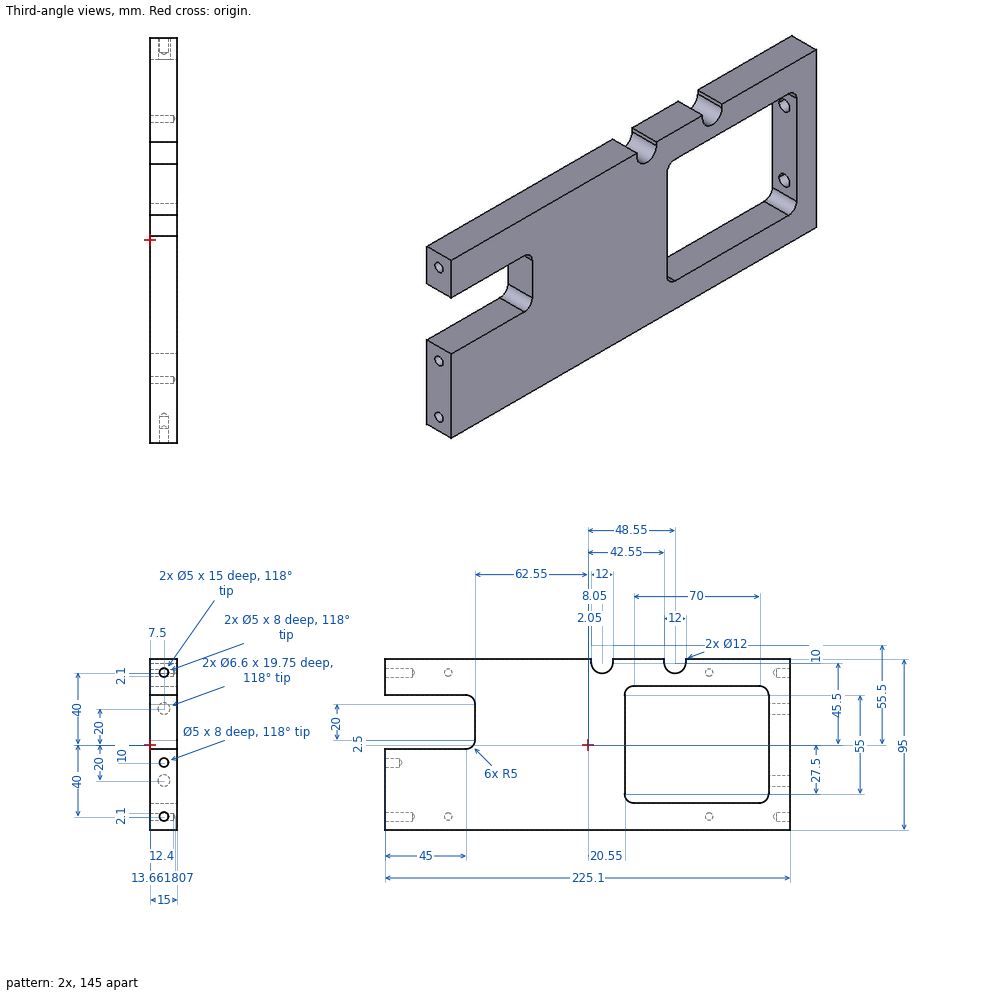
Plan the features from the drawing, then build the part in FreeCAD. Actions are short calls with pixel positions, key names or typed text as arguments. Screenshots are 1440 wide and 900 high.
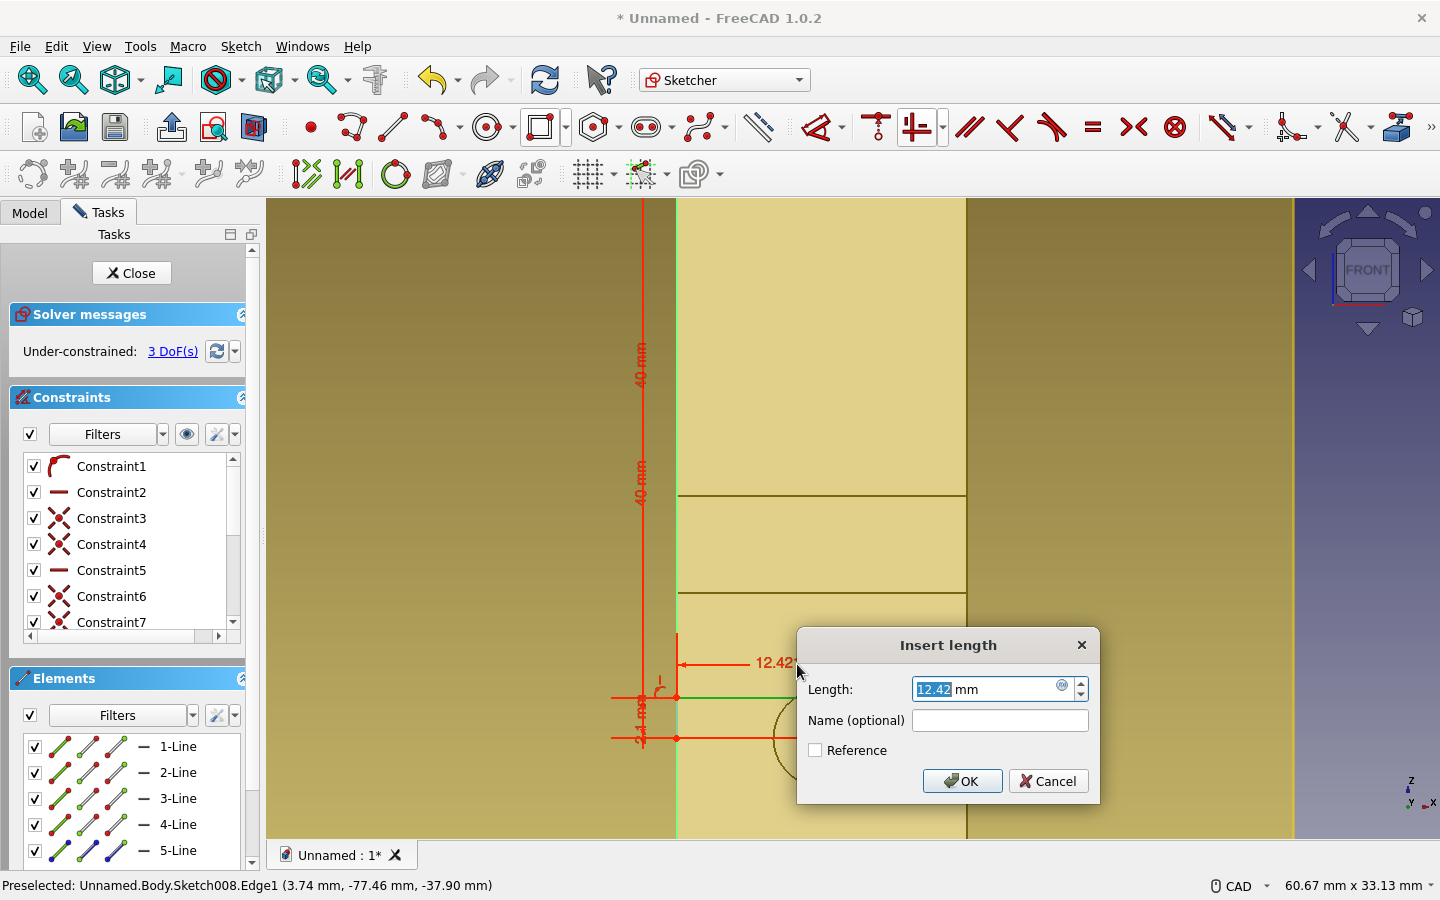
text(12.4)
key(Return)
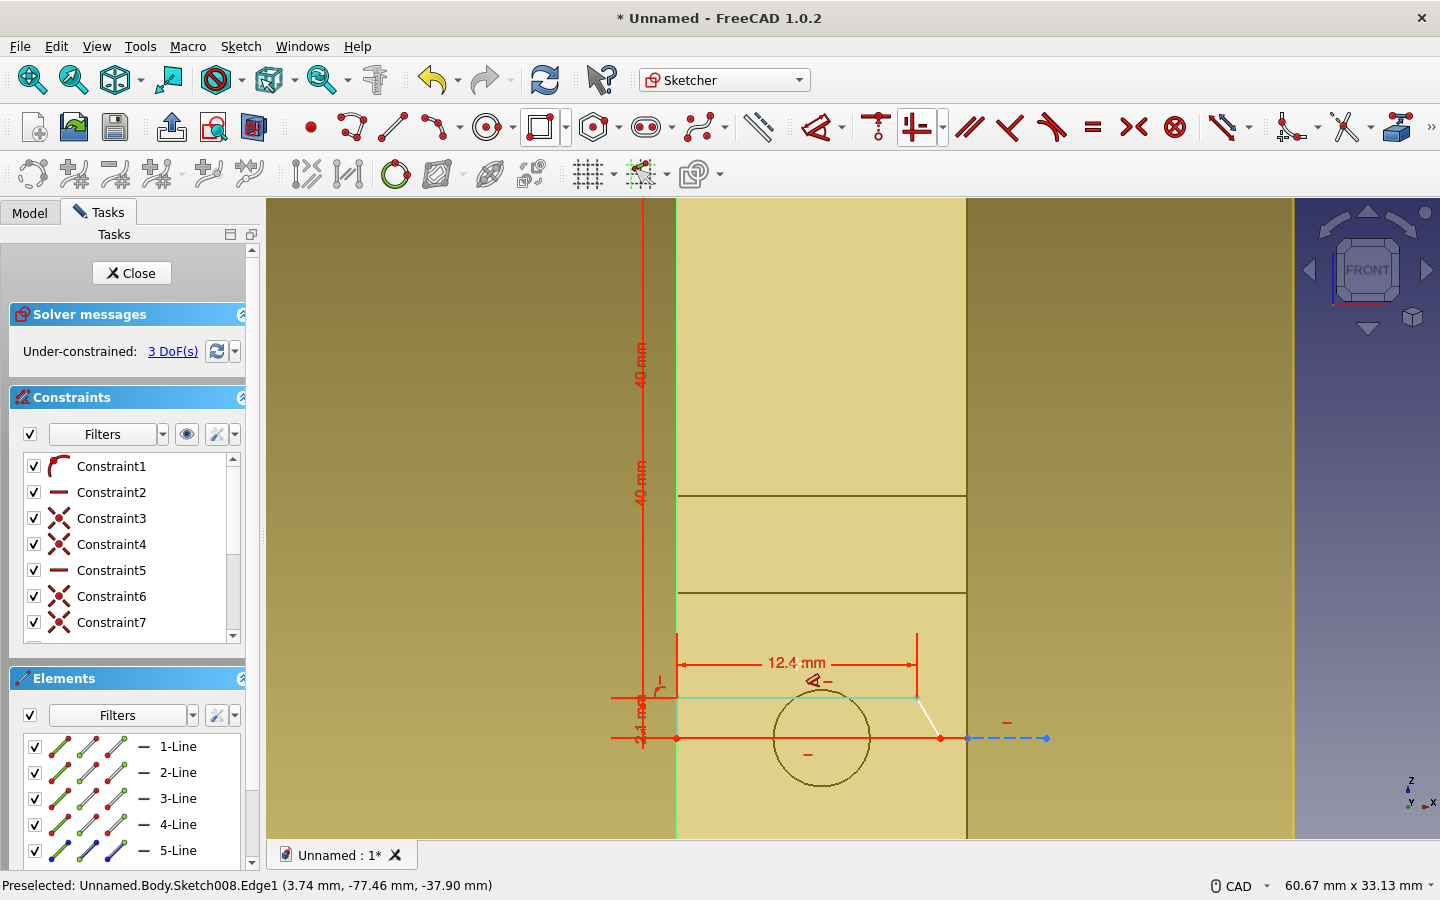
click(861, 738)
click(809, 772)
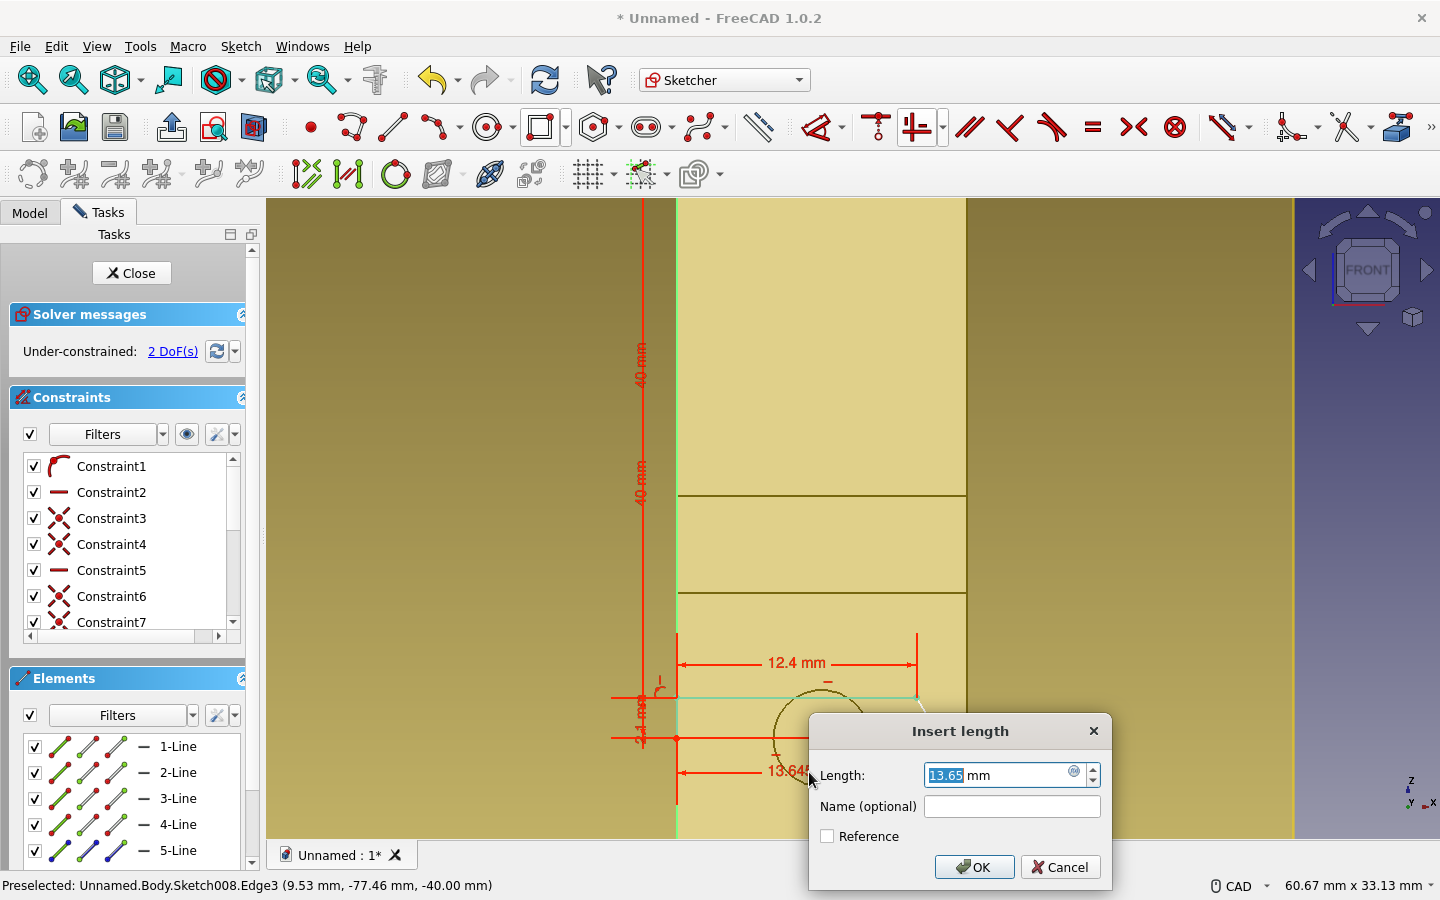
text(13.661807)
key(Return)
key(Escape)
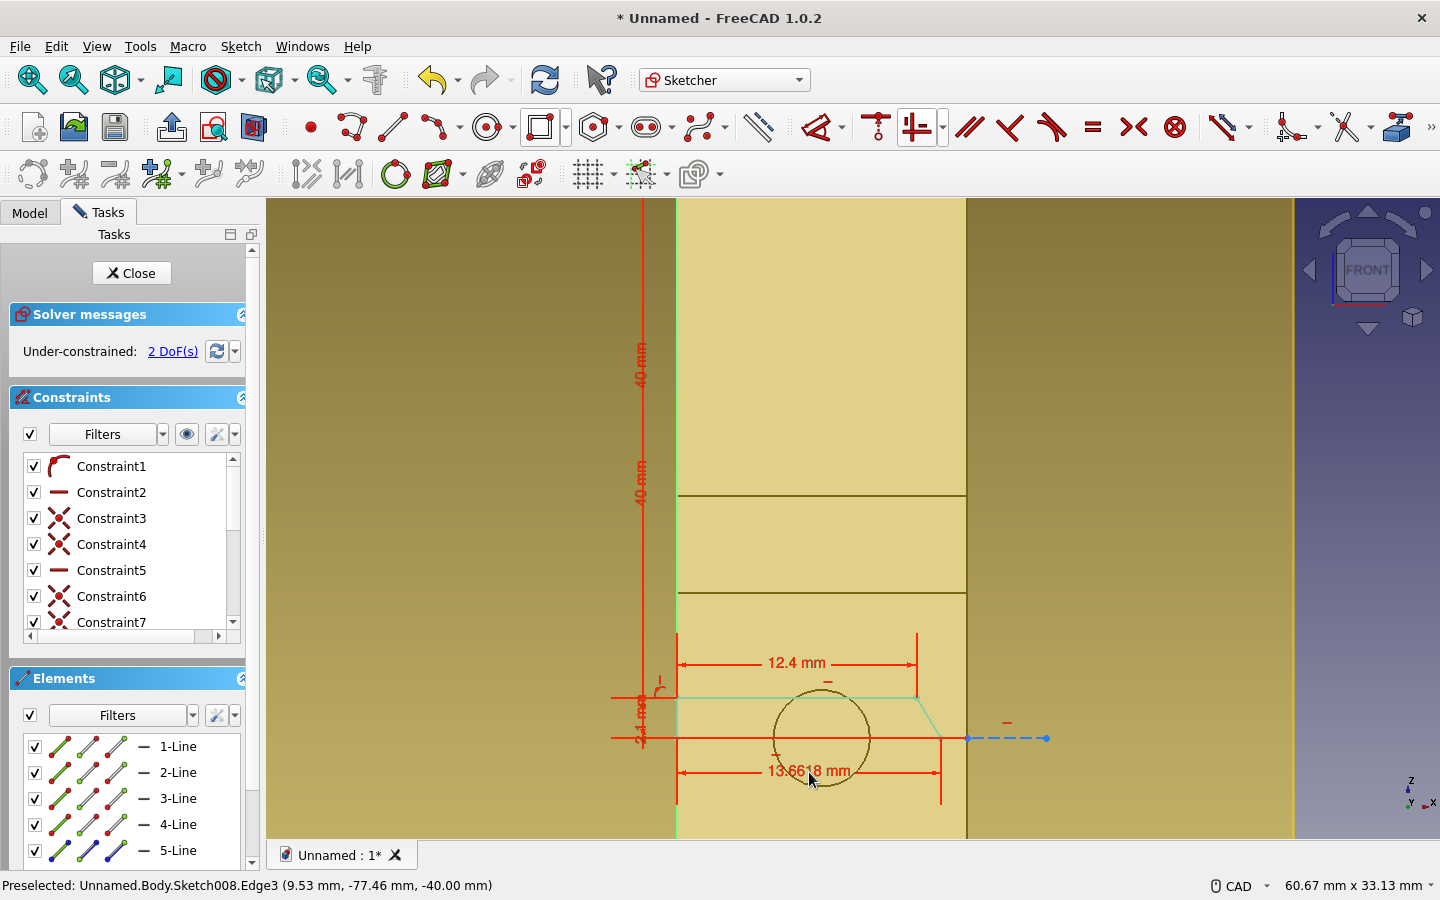
click(132, 273)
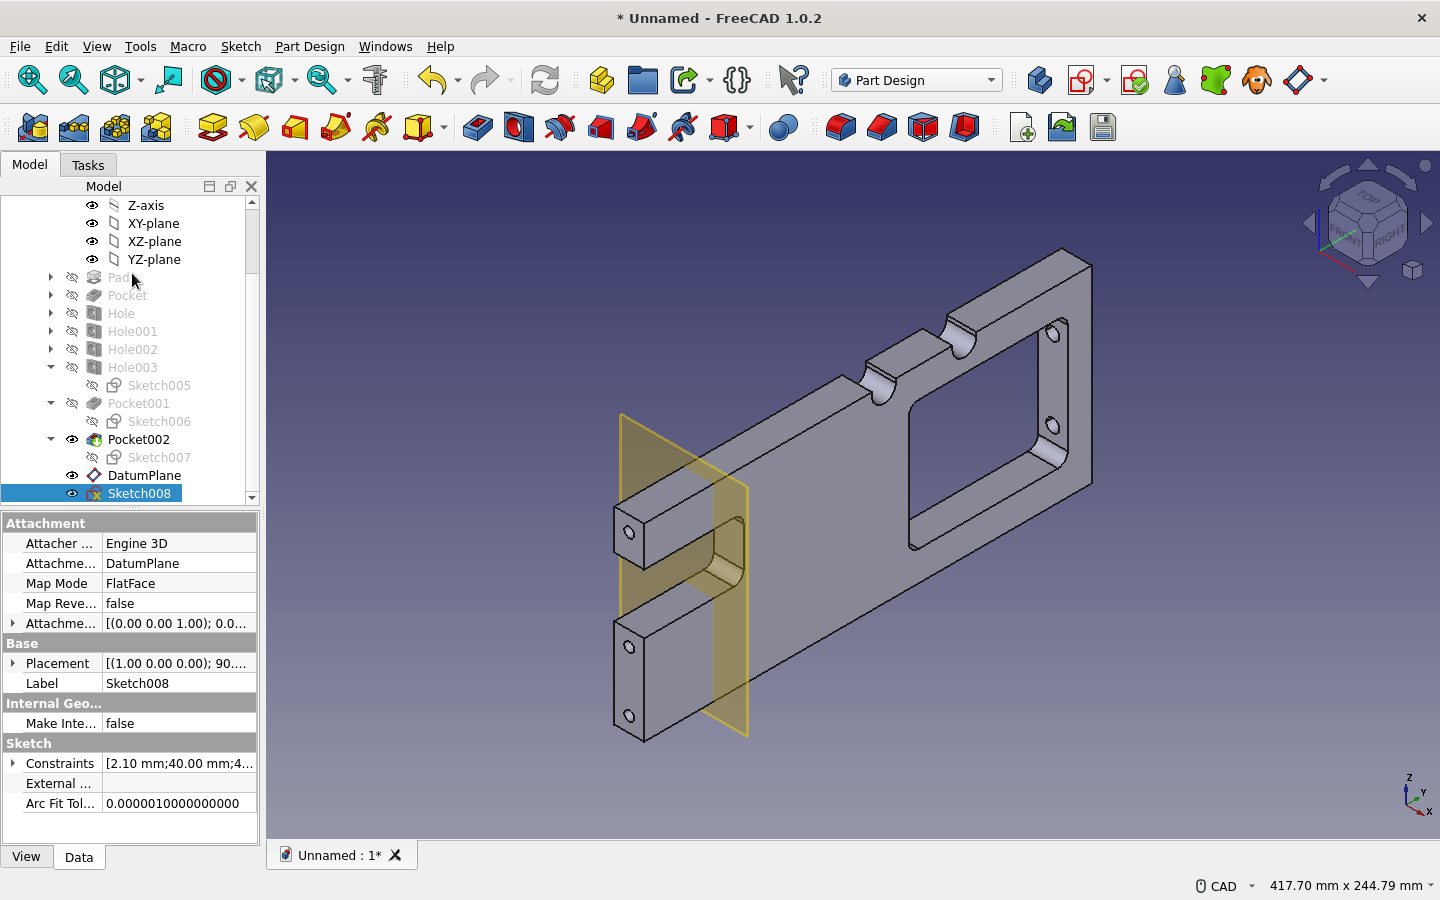
click(560, 128)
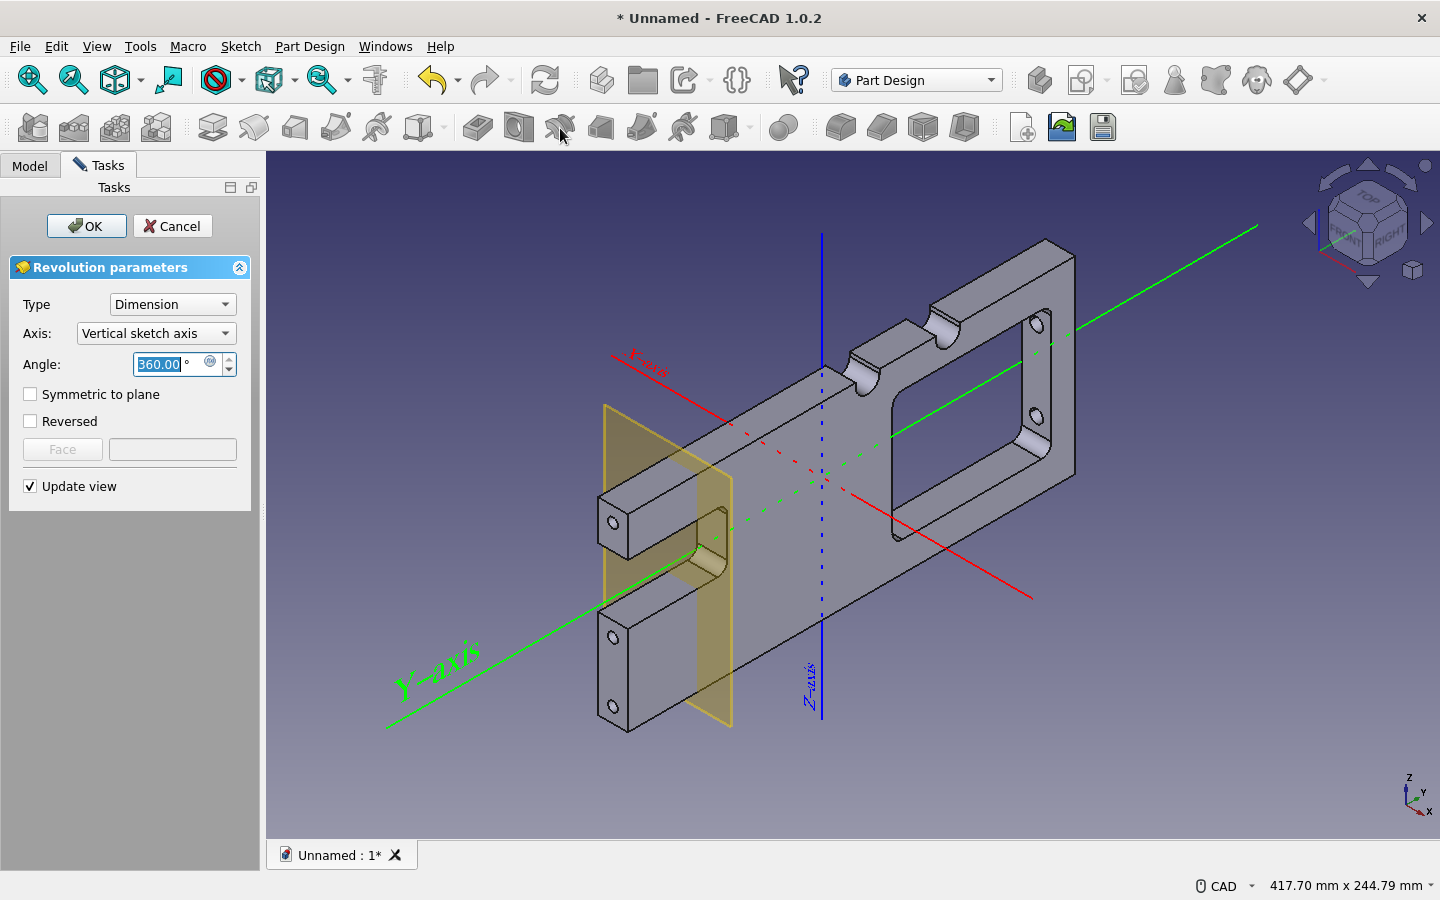
click(157, 334)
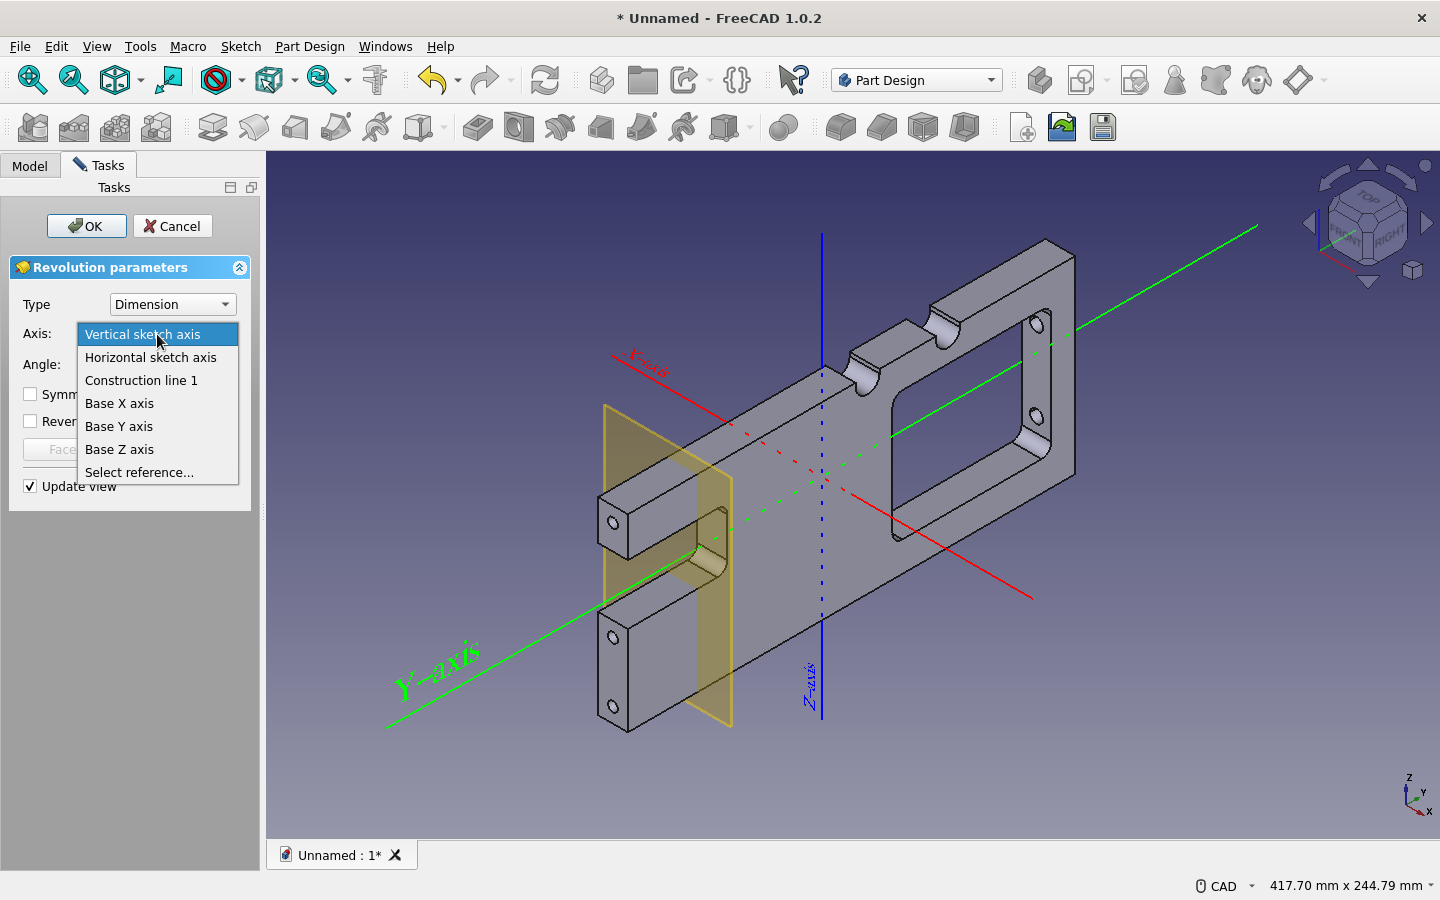
click(156, 380)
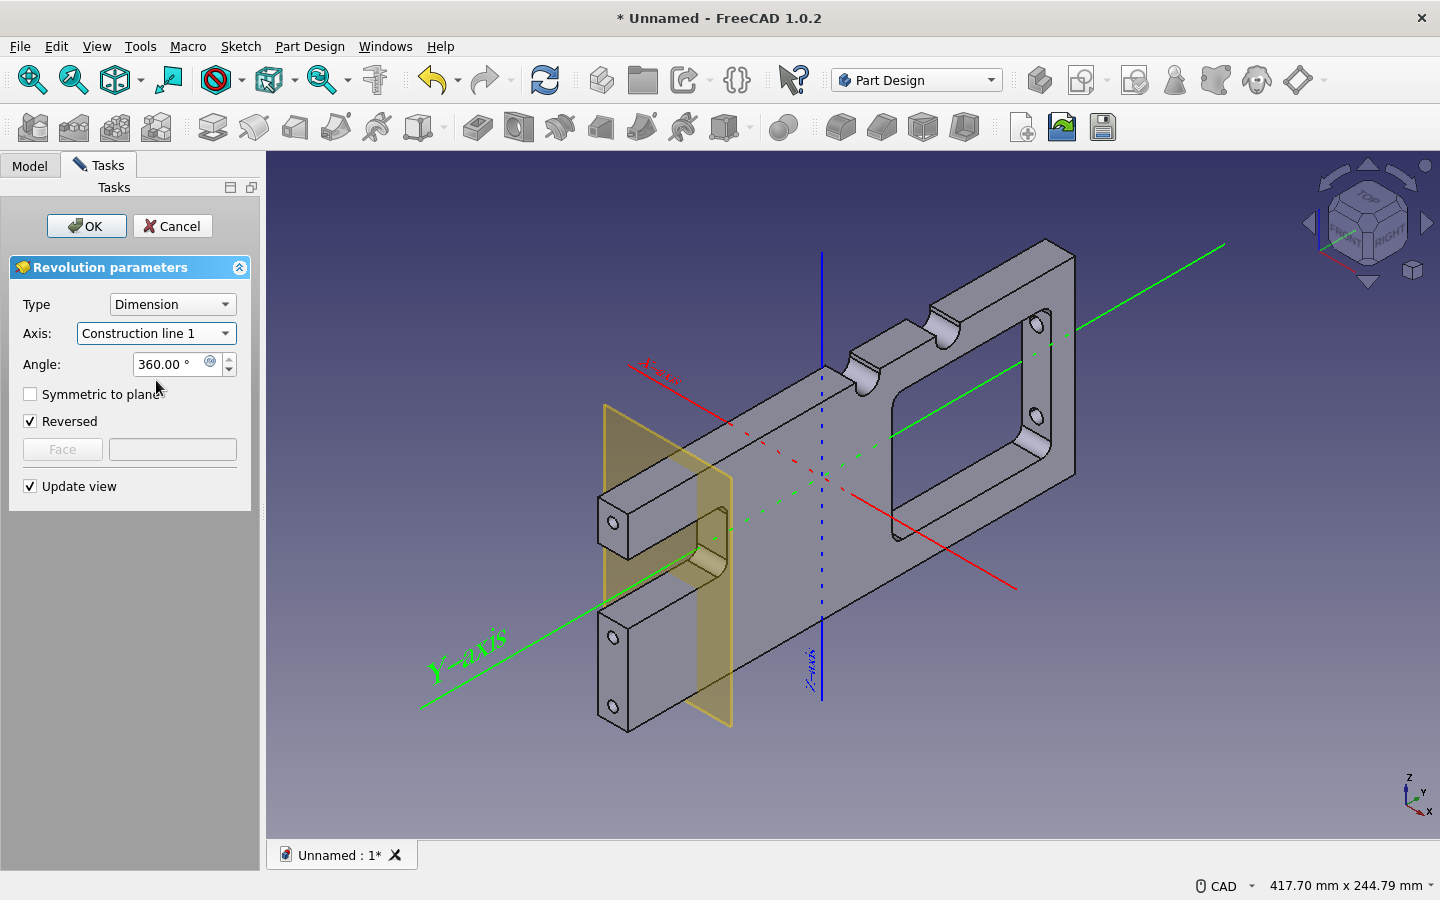
click(87, 226)